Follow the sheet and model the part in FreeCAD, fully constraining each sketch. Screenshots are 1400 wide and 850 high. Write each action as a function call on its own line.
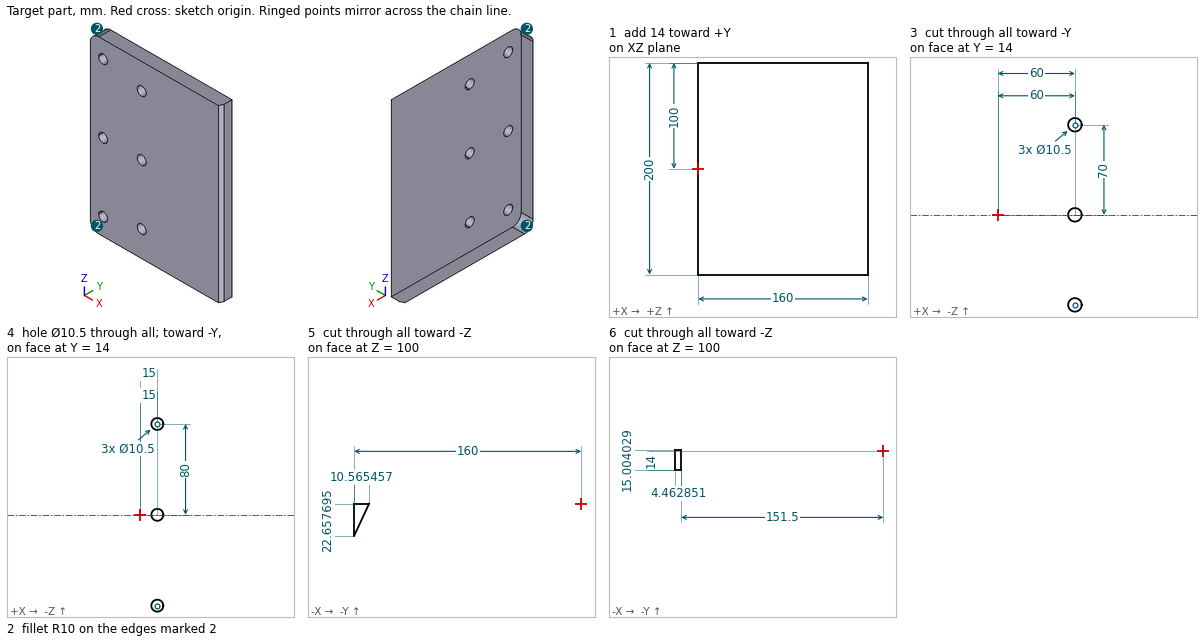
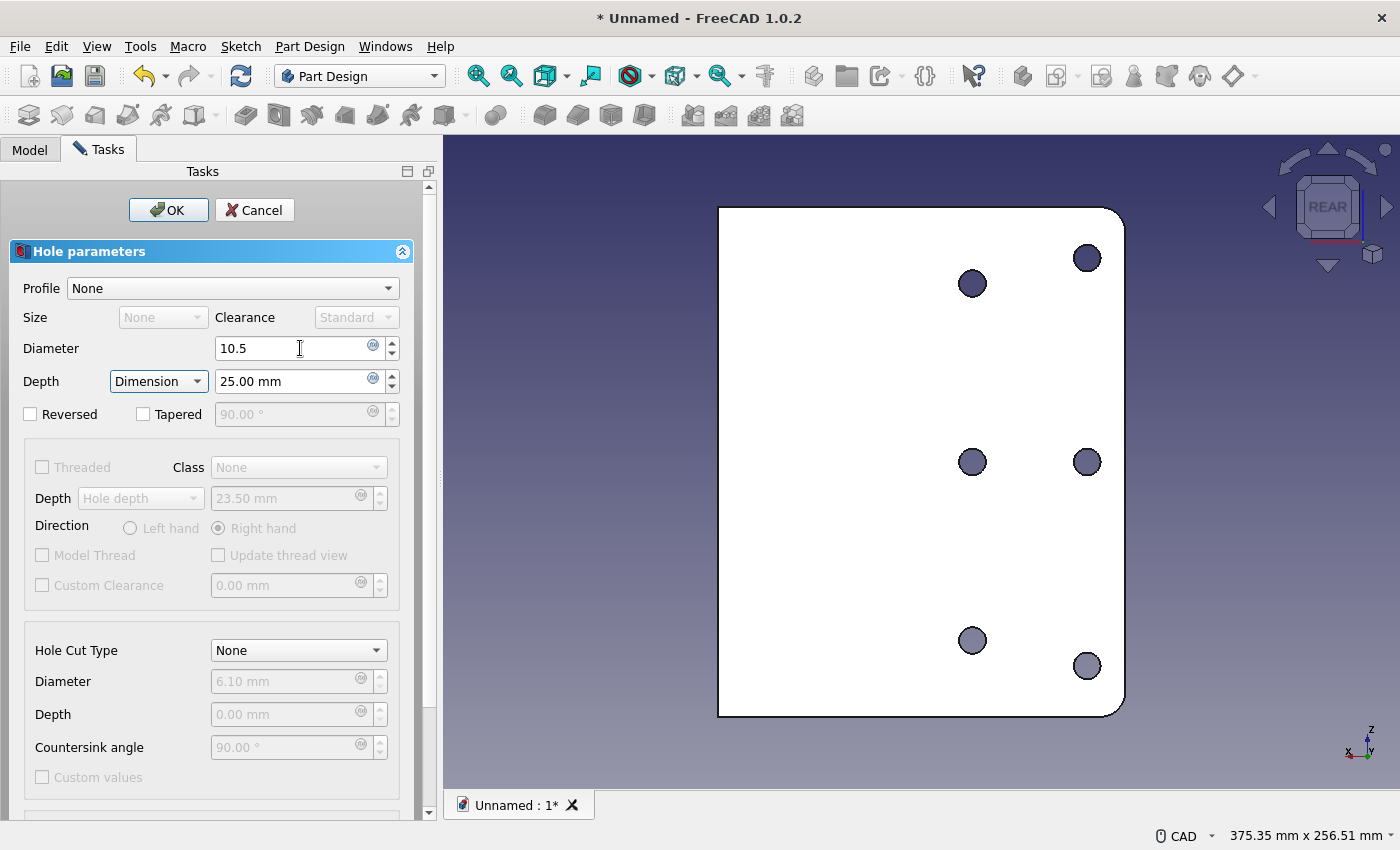
click(160, 382)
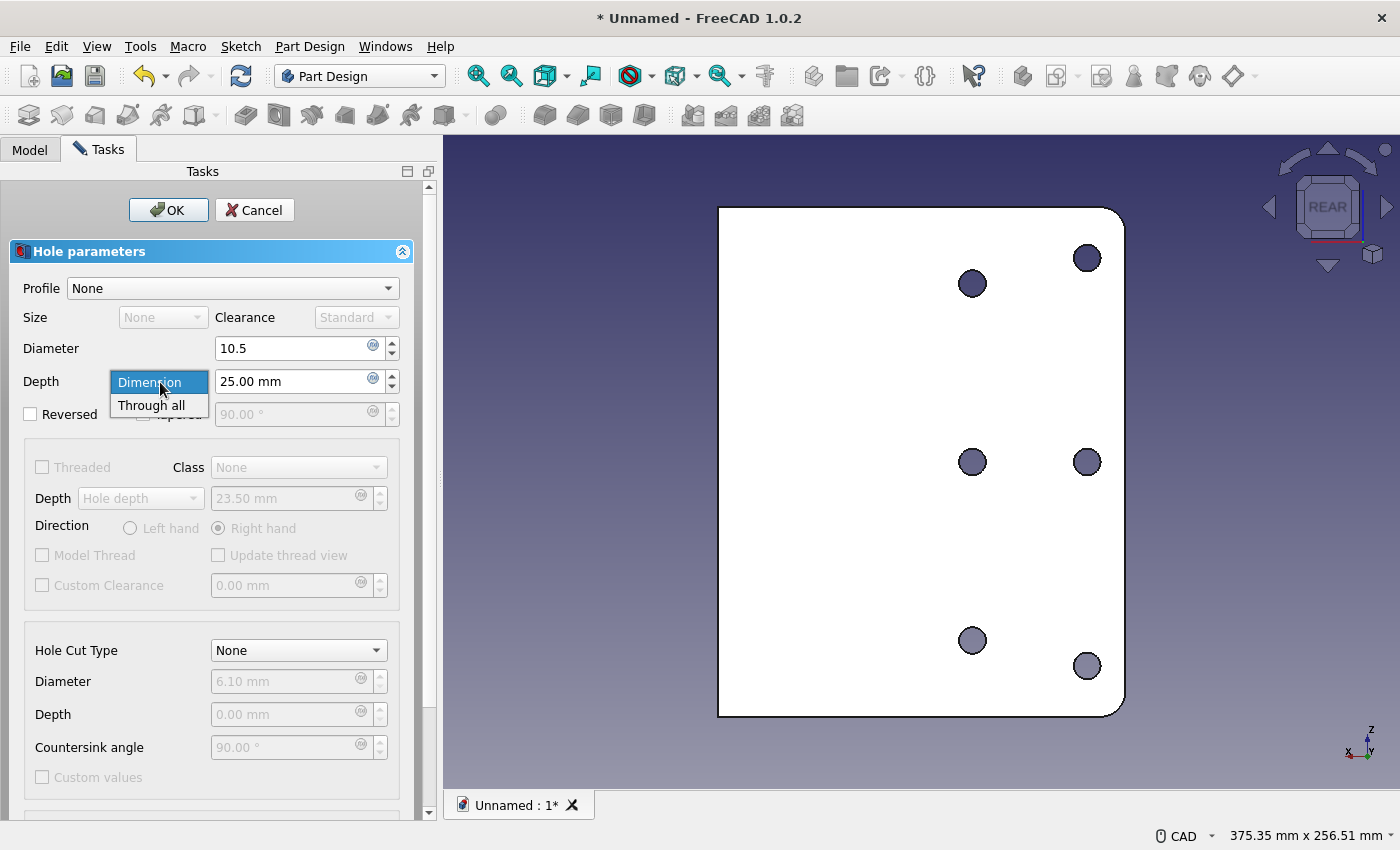
click(158, 406)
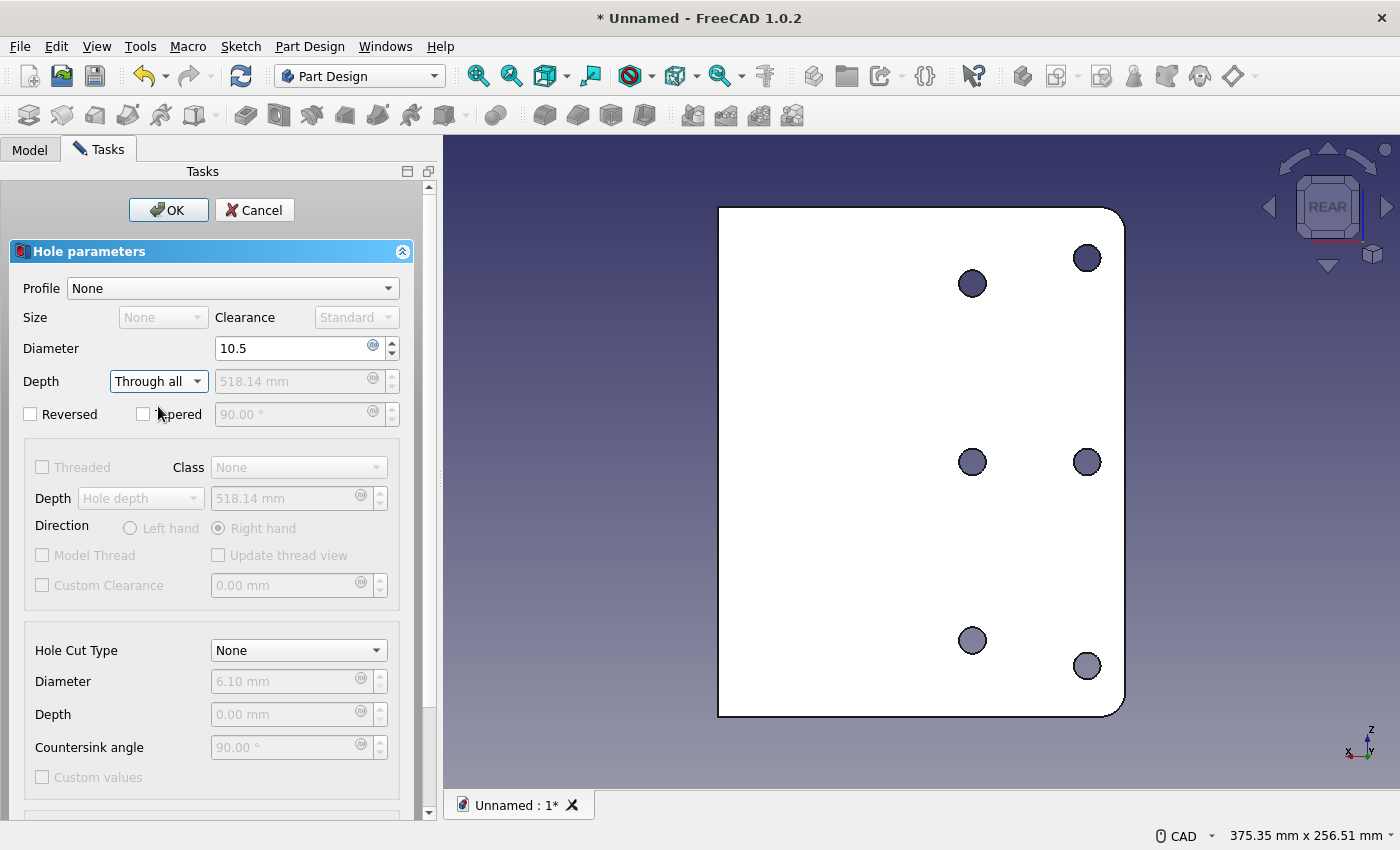
click(169, 210)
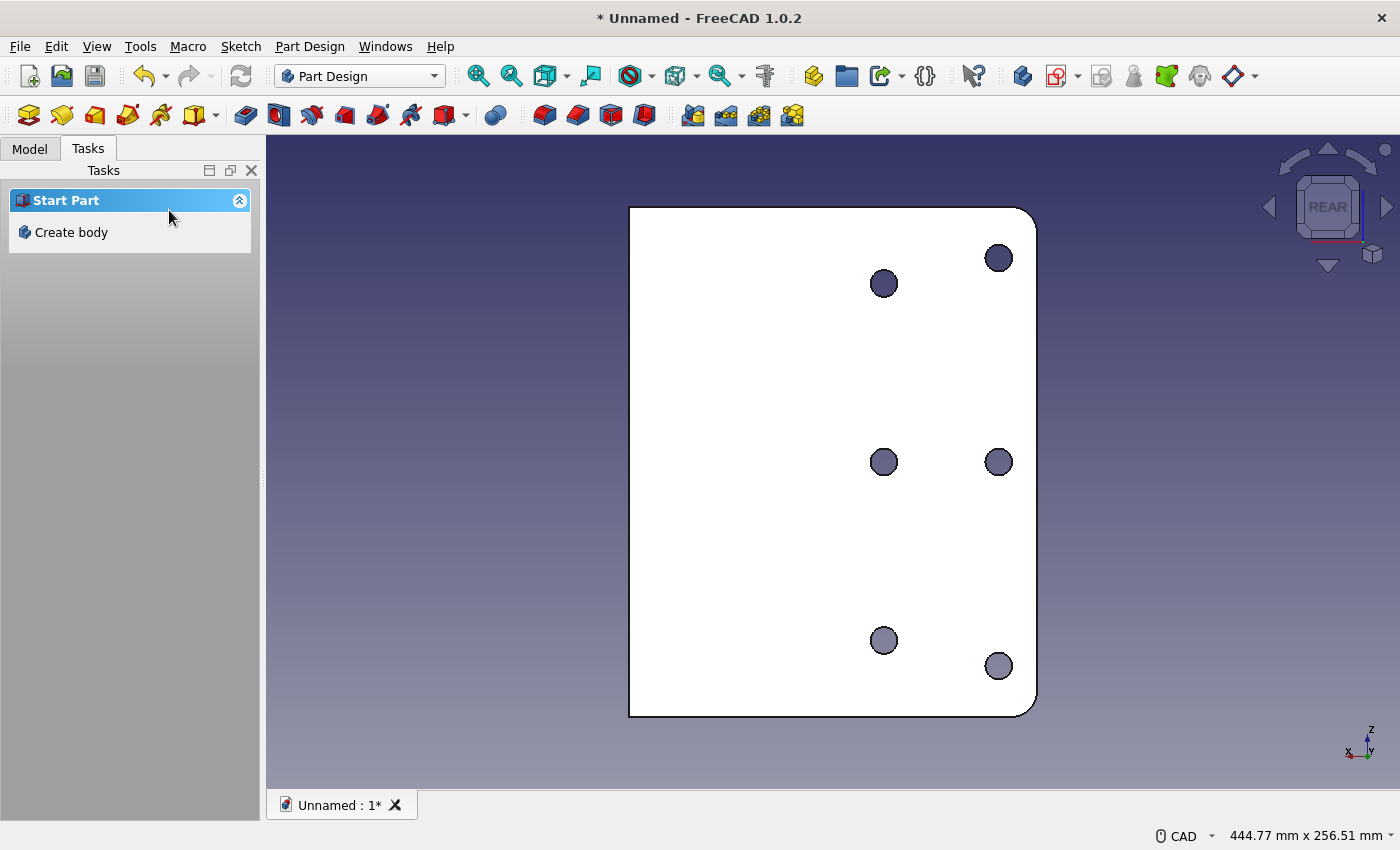
key(0)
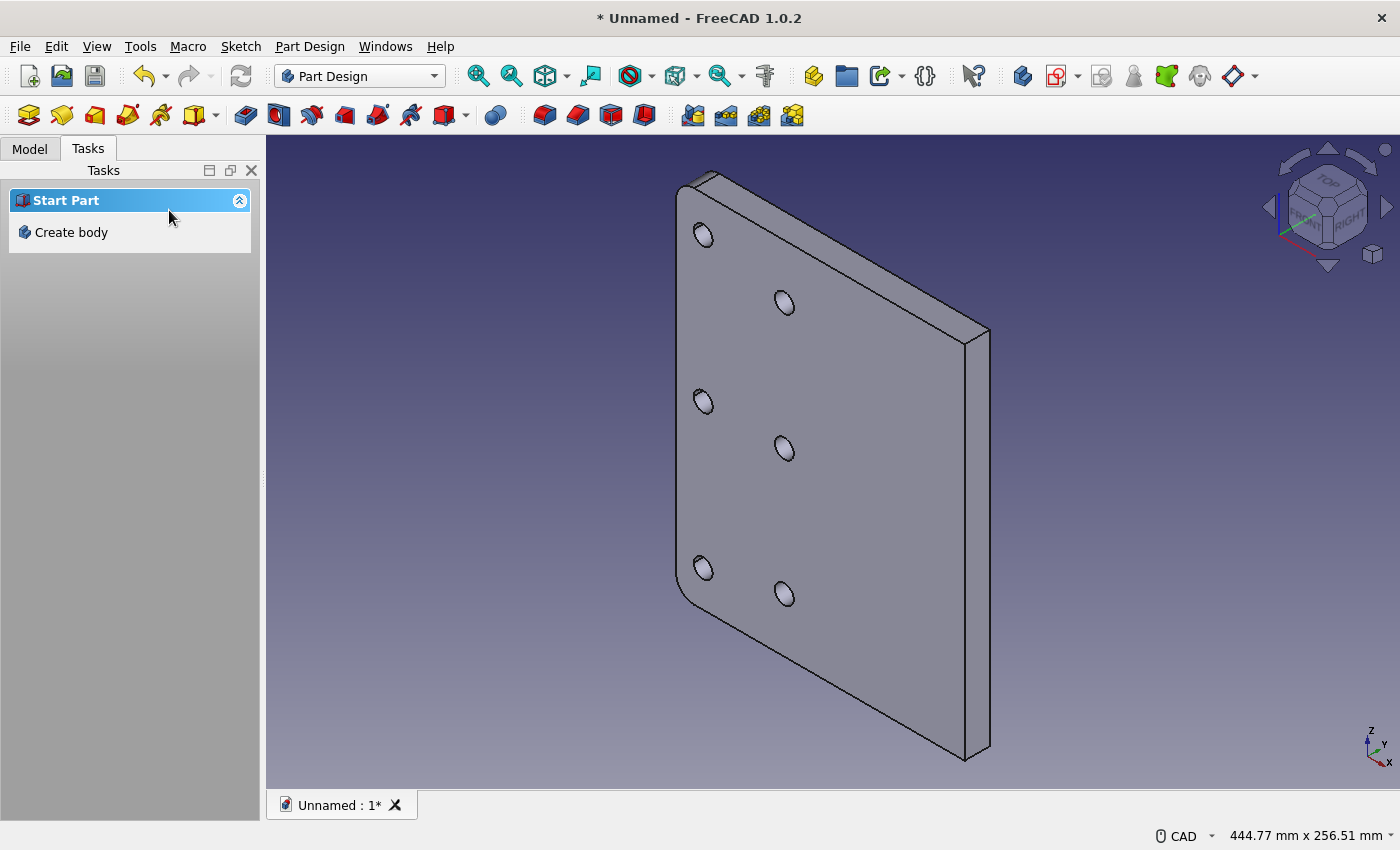
click(958, 325)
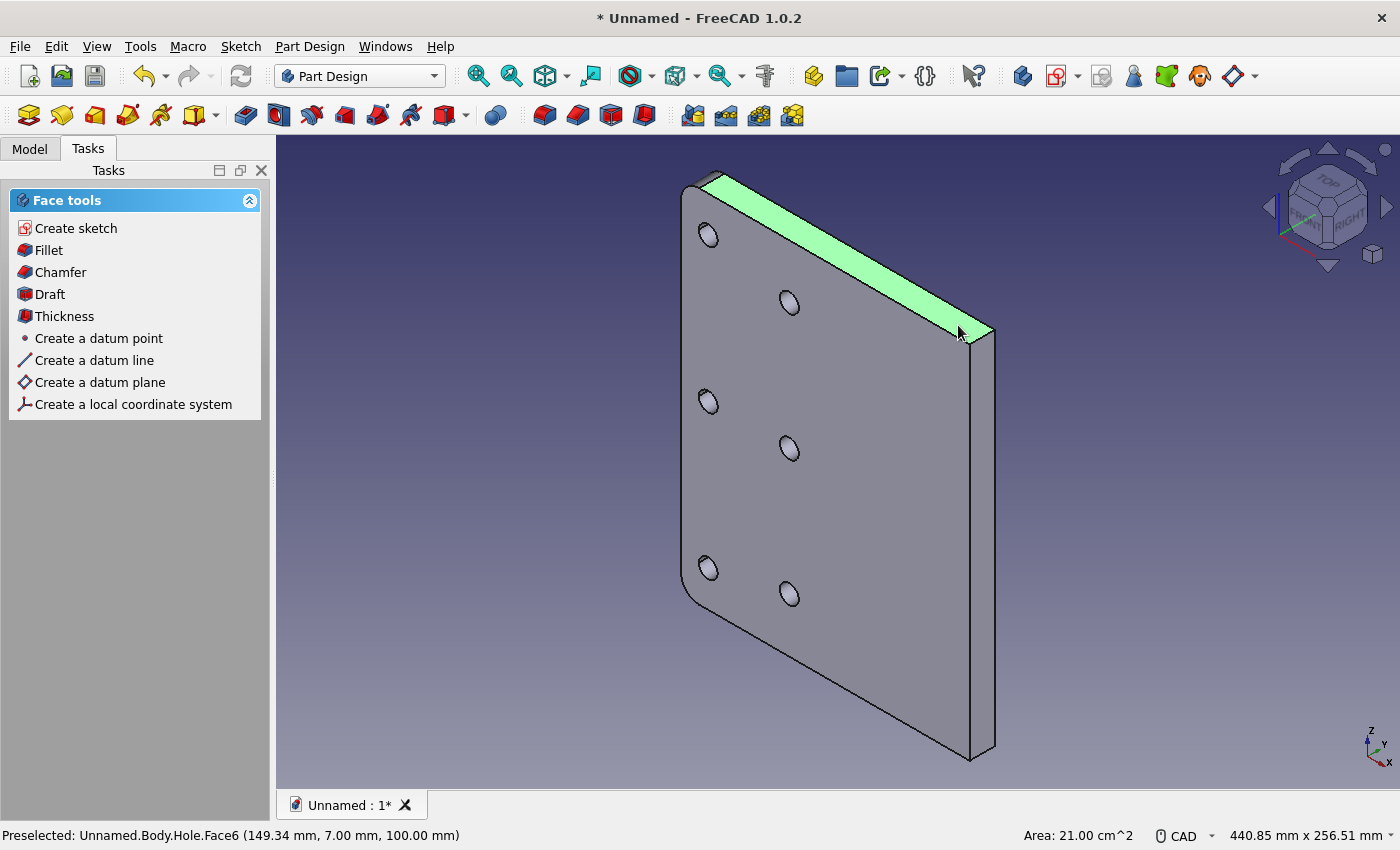
click(1056, 76)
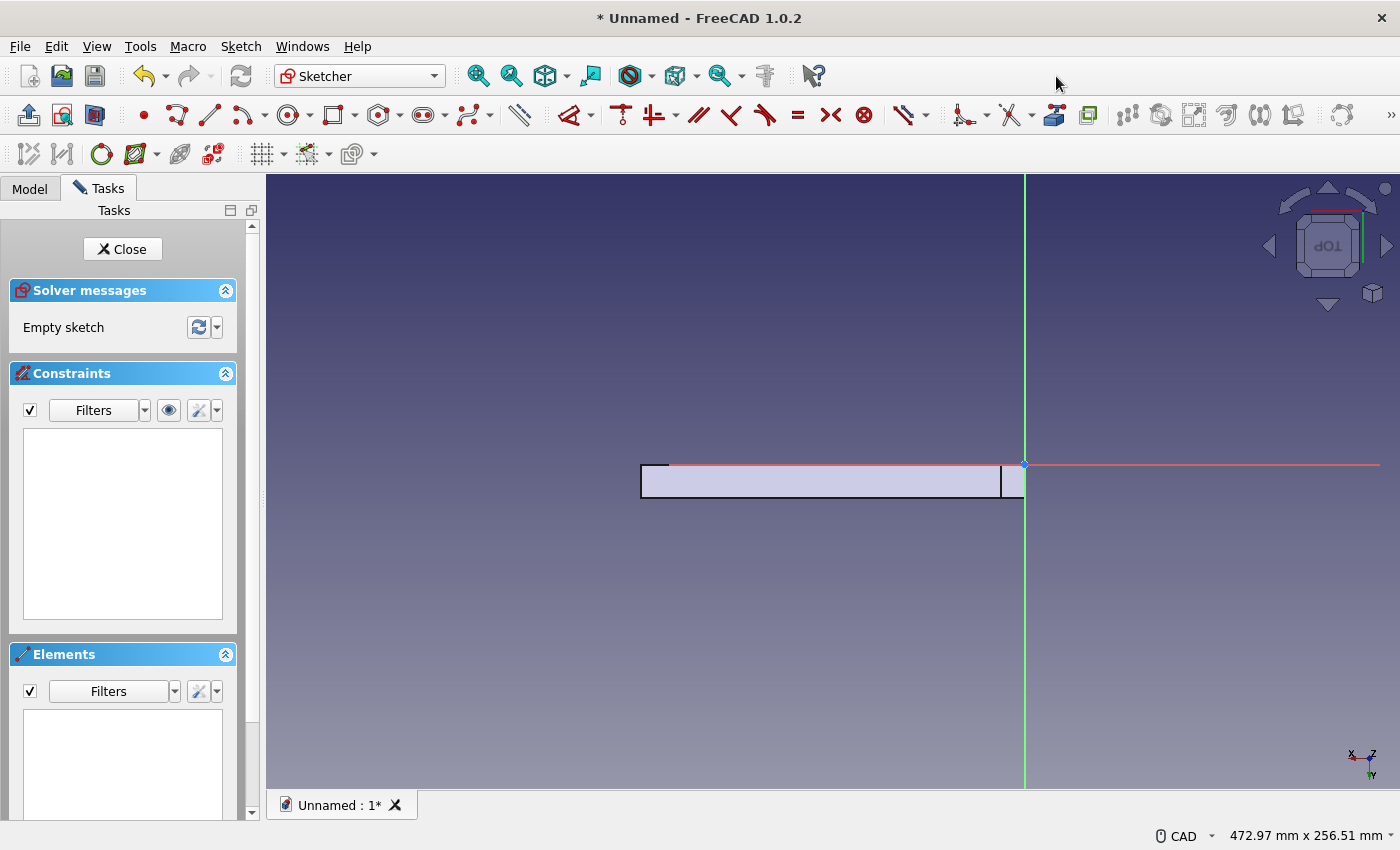
scroll(637, 494, up, 10)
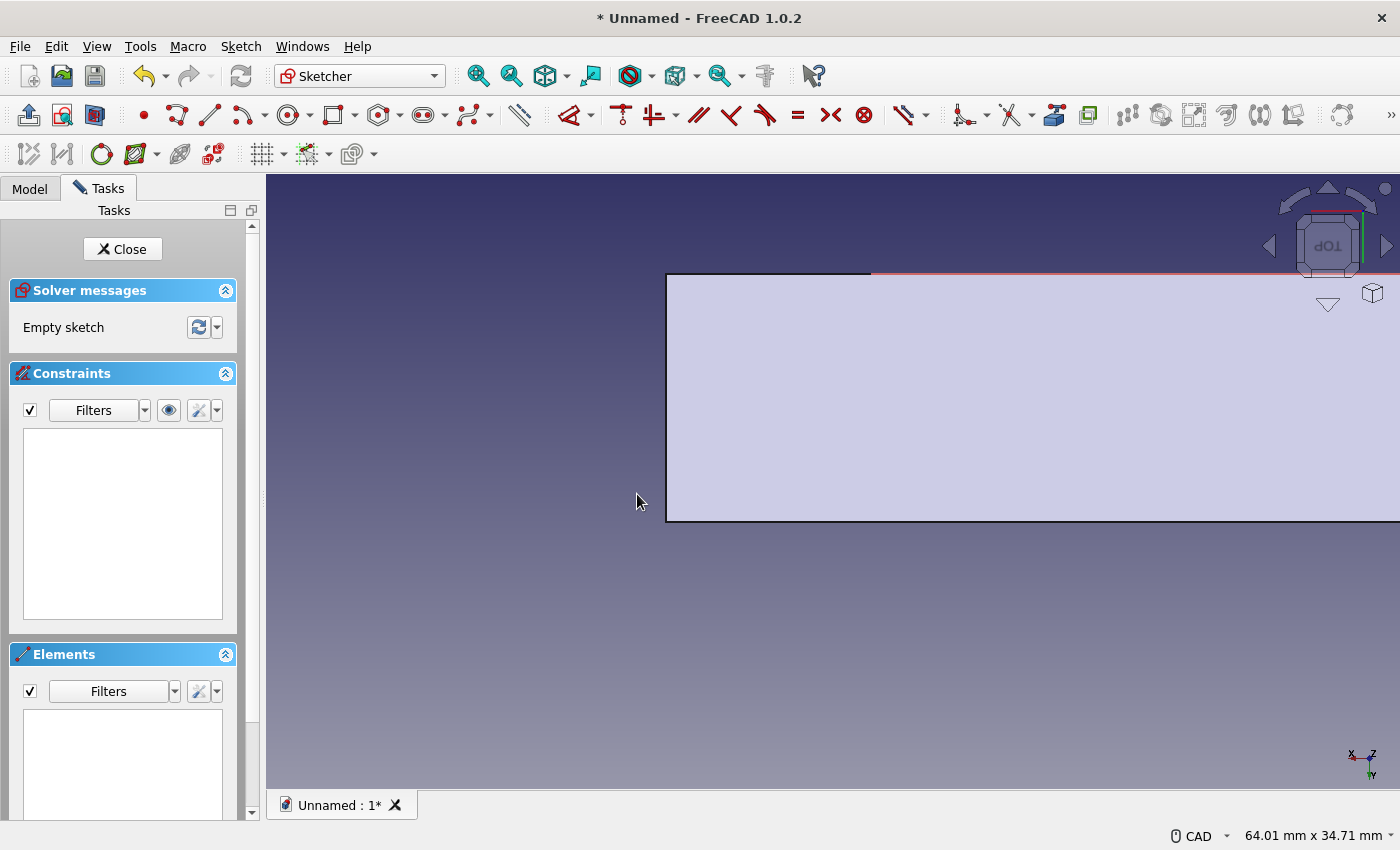
click(177, 116)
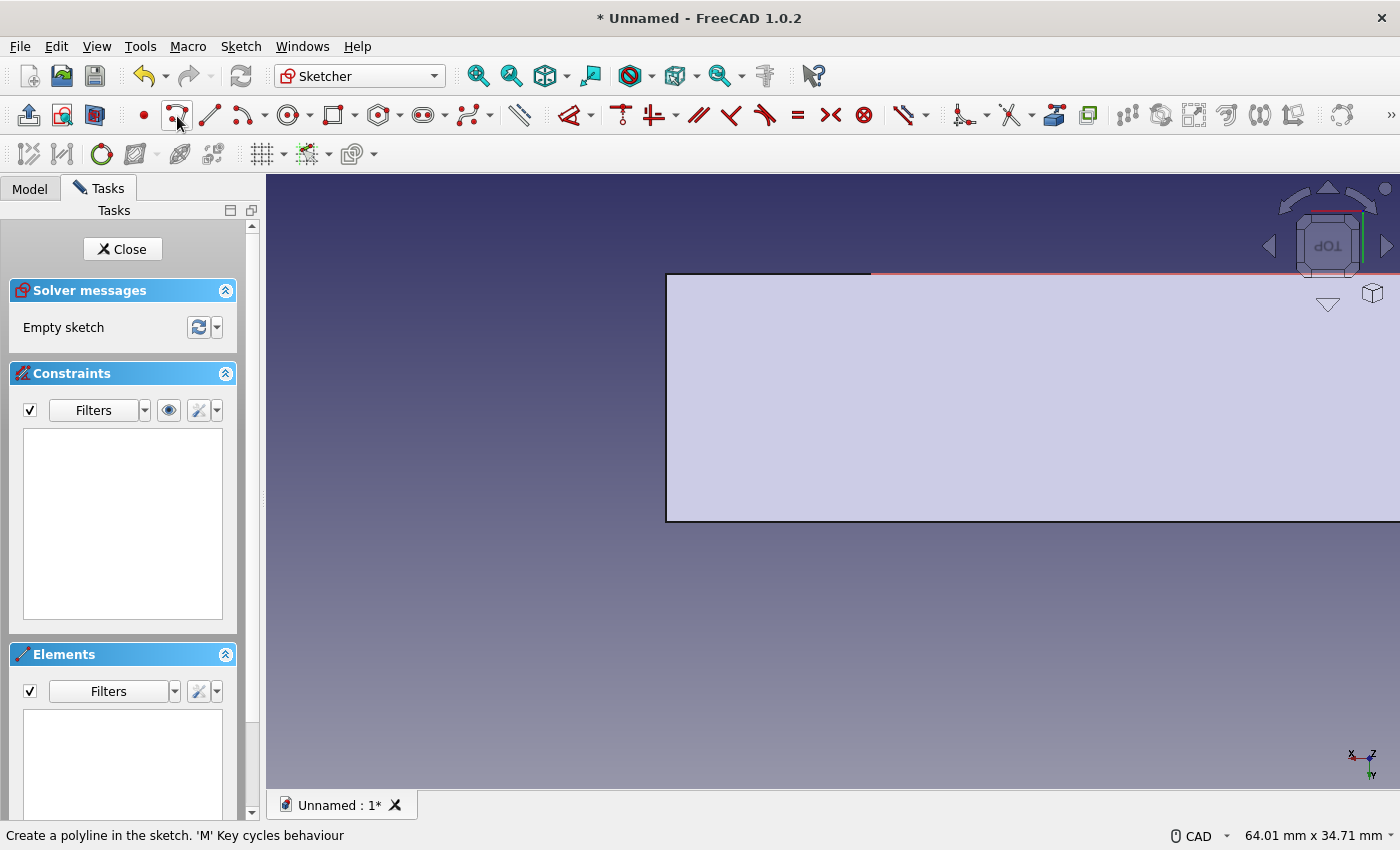
click(853, 274)
click(666, 283)
click(666, 676)
click(853, 275)
key(Escape)
key(Escape)